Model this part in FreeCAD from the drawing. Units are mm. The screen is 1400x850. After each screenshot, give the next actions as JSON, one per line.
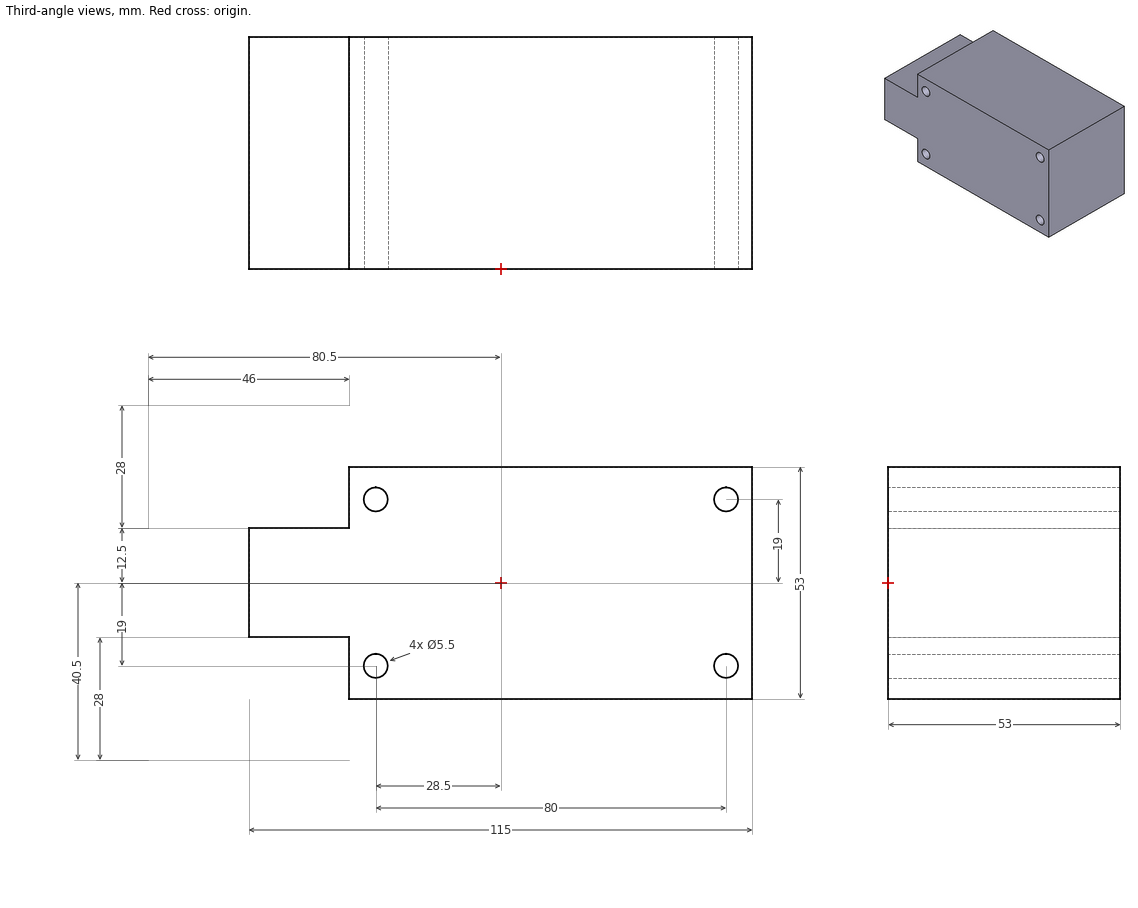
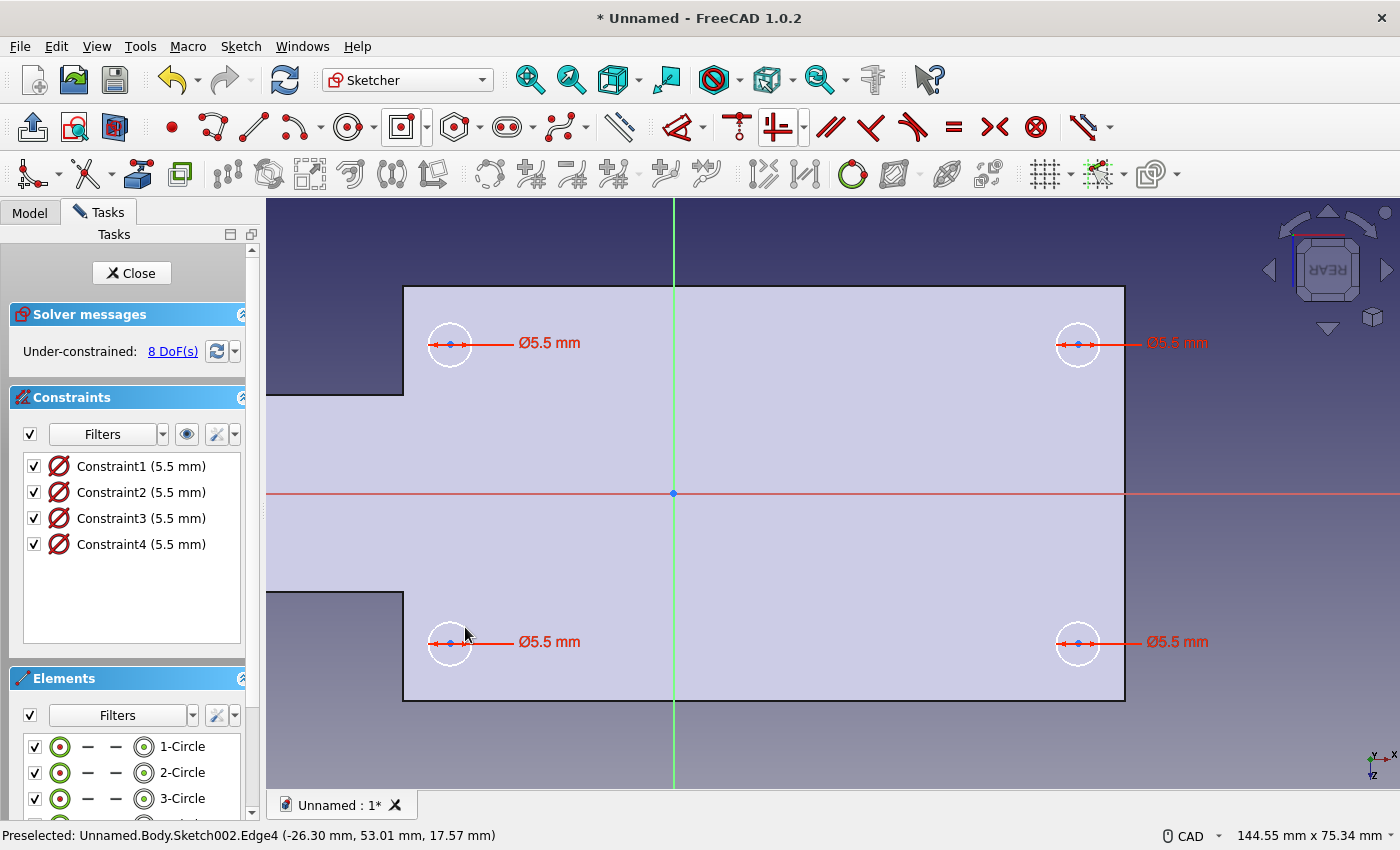
{"action": "left_click", "coordinate": [676, 128]}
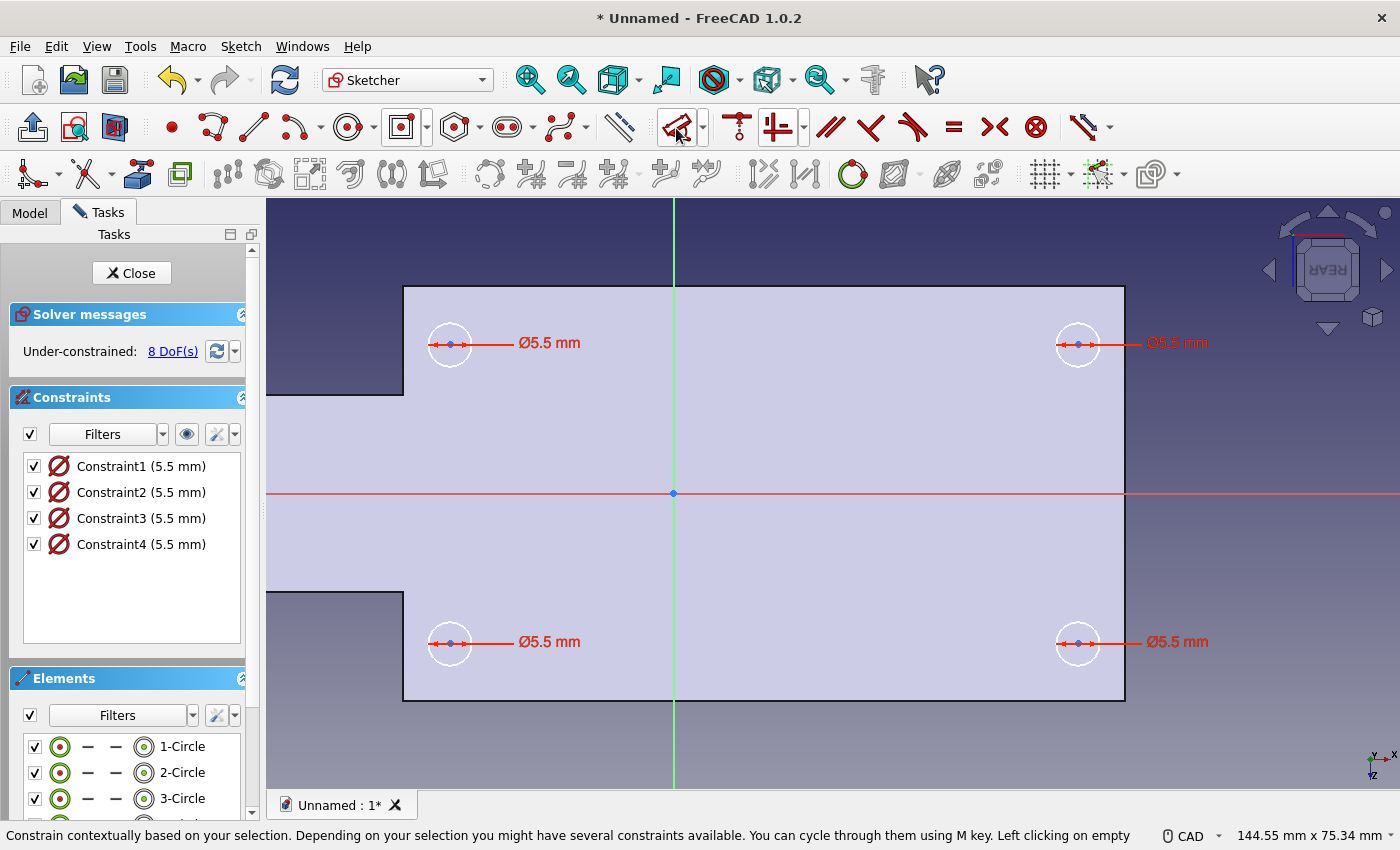
{"action": "left_click", "coordinate": [450, 345]}
{"action": "left_click", "coordinate": [416, 419]}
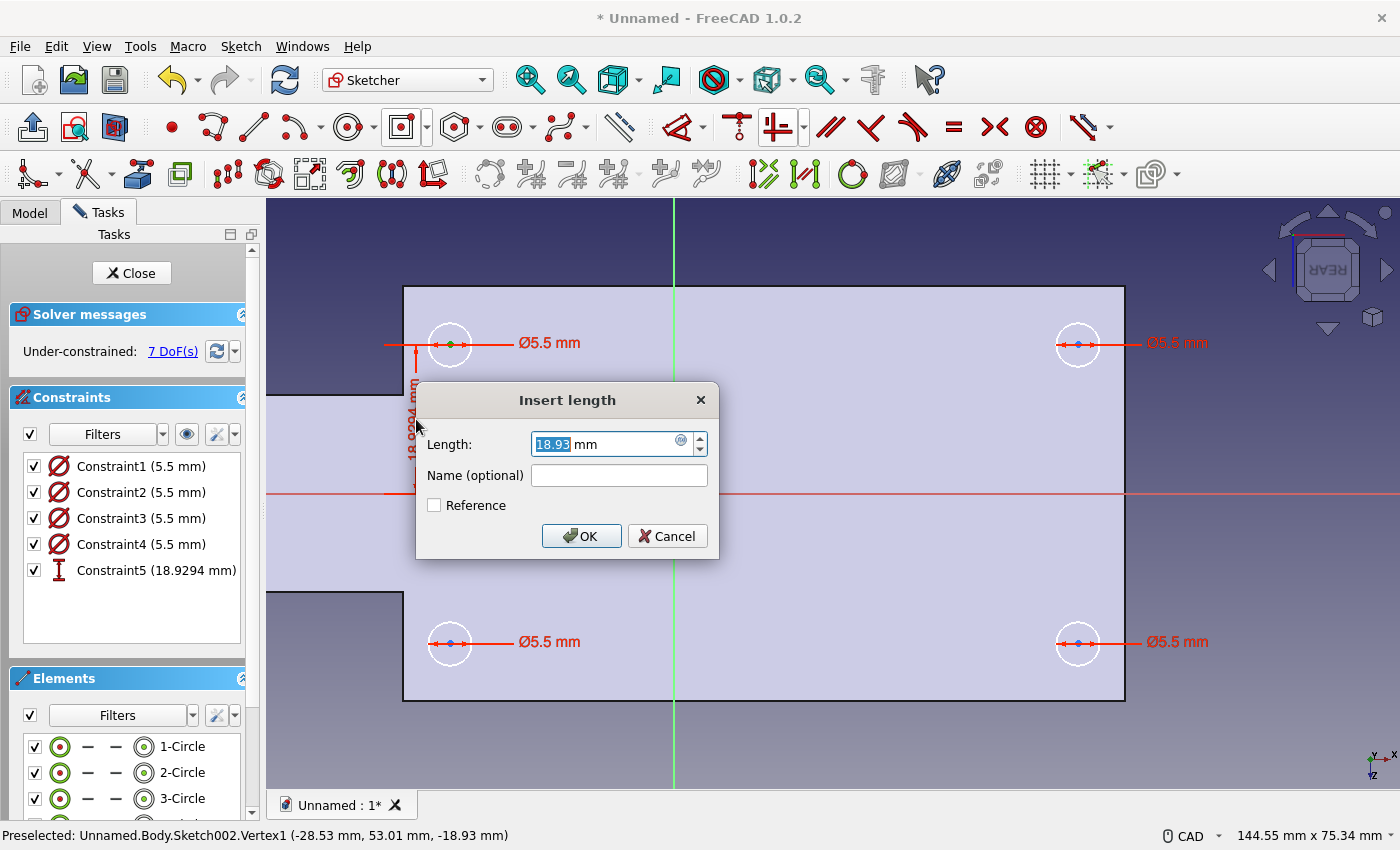
{"action": "type", "text": "19"}
{"action": "key", "text": "Return"}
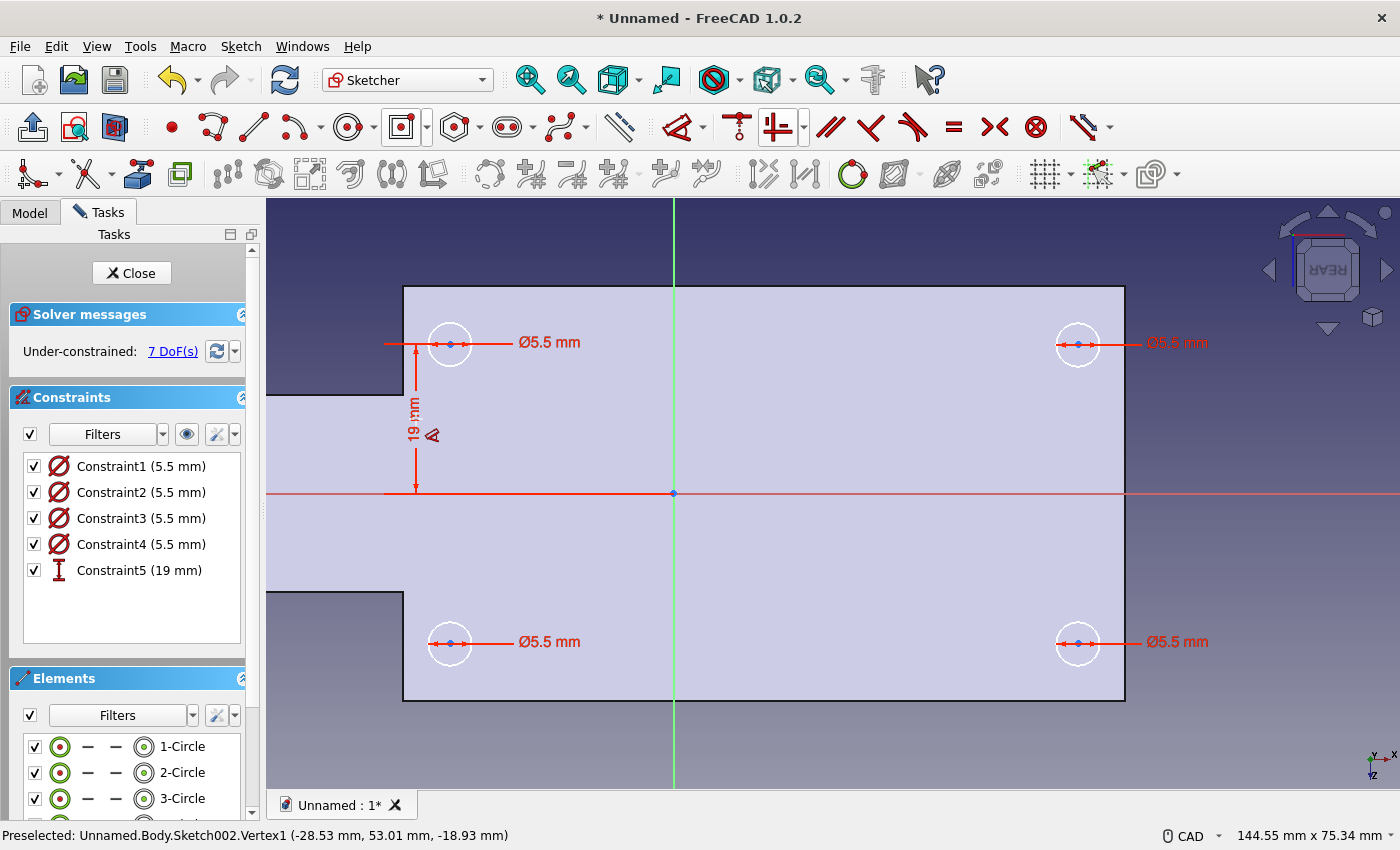
{"action": "left_click", "coordinate": [1078, 345]}
{"action": "left_click", "coordinate": [1112, 419]}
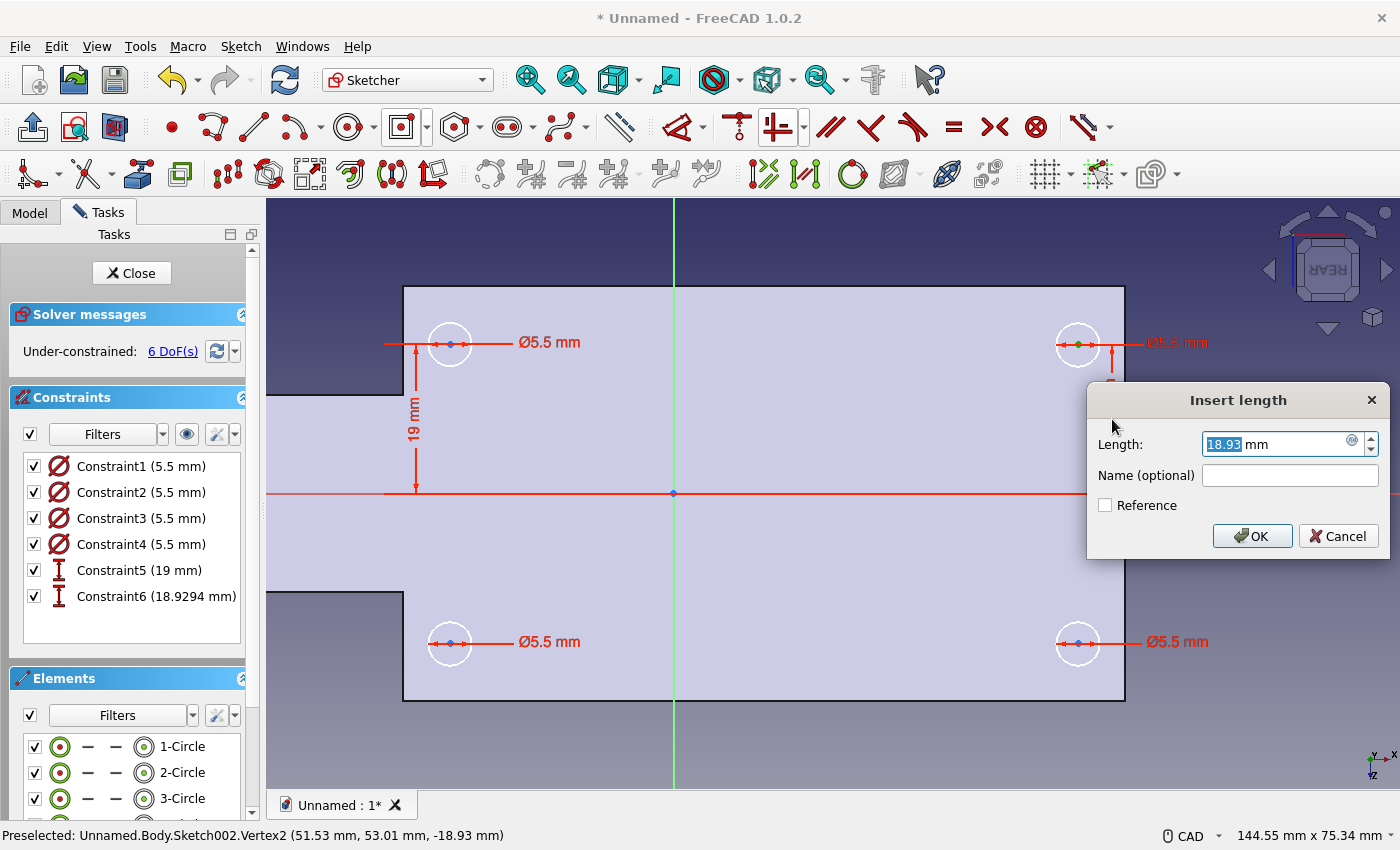
{"action": "type", "text": "19"}
{"action": "key", "text": "Return"}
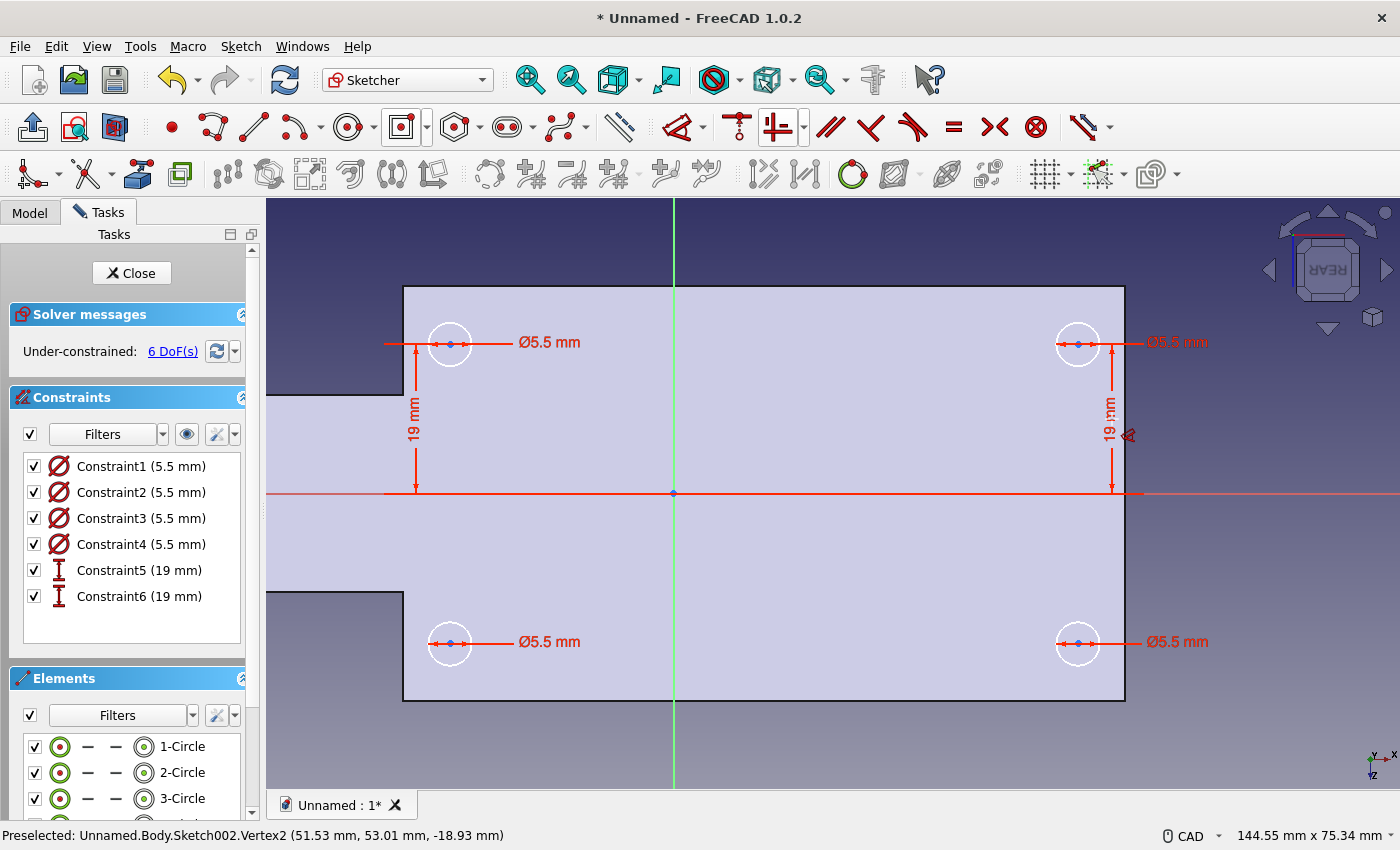
{"action": "left_click", "coordinate": [1078, 644]}
{"action": "left_click", "coordinate": [1112, 569]}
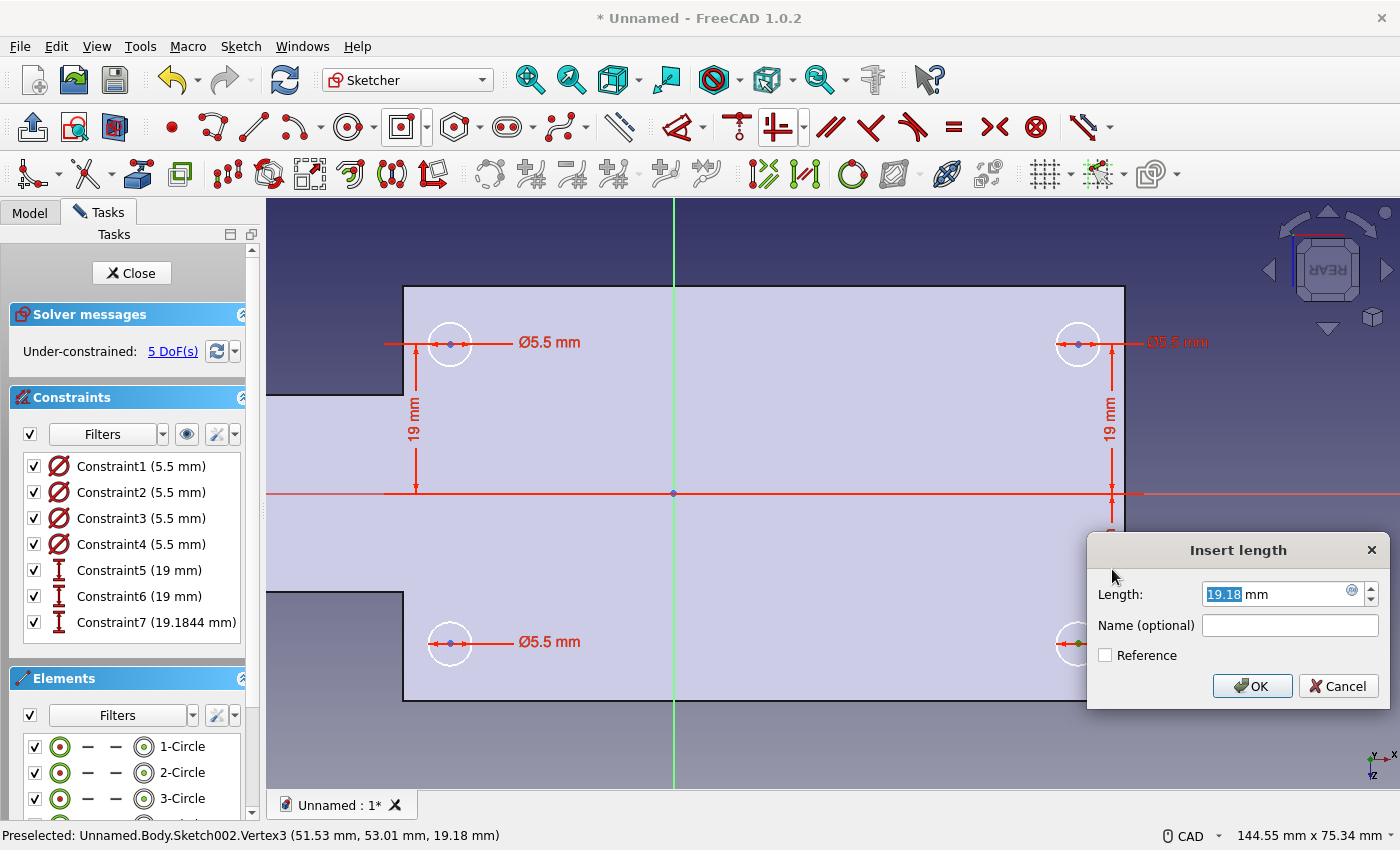
{"action": "type", "text": "19"}
{"action": "key", "text": "Return"}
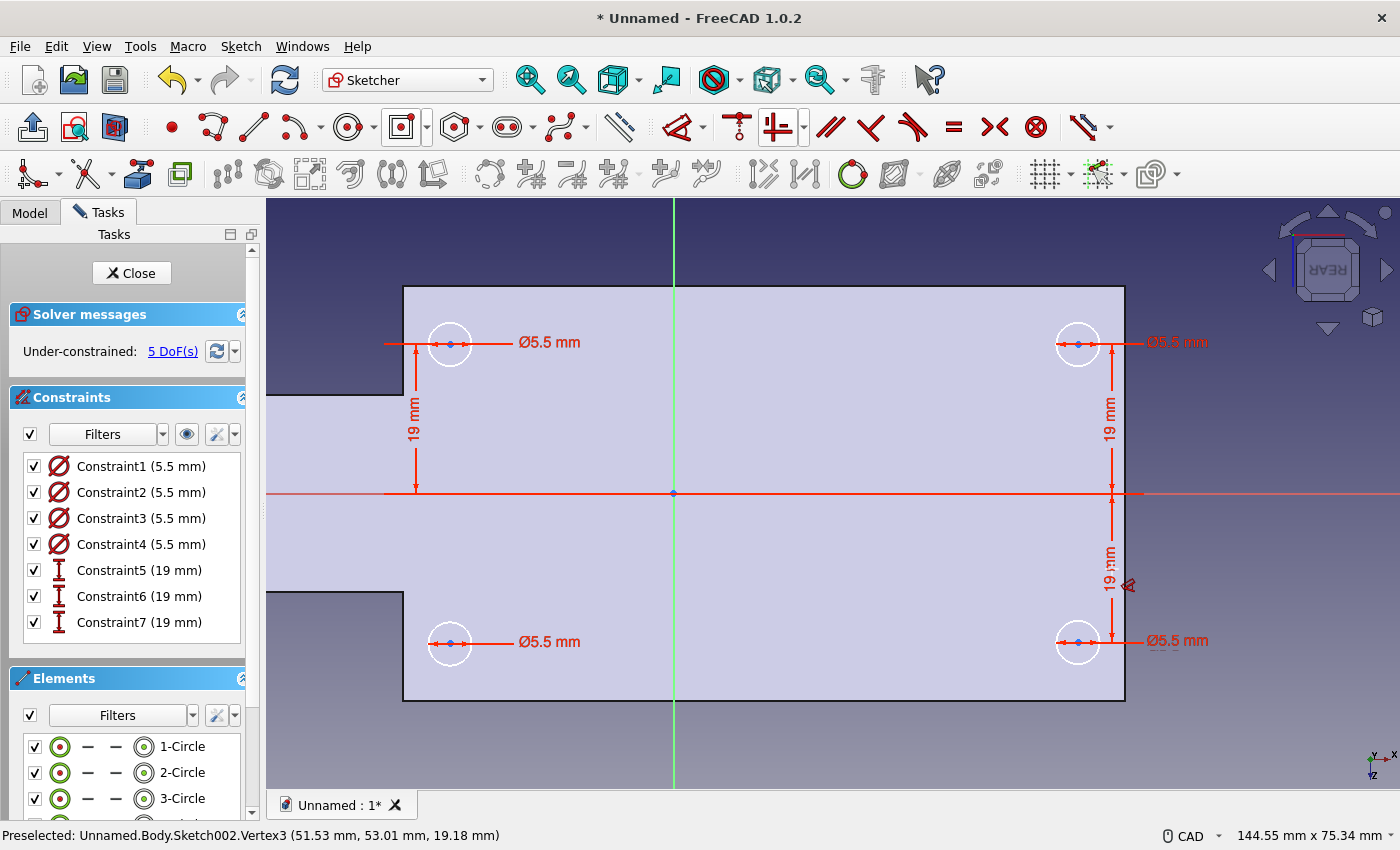
{"action": "left_click", "coordinate": [450, 644]}
{"action": "left_click", "coordinate": [416, 569]}